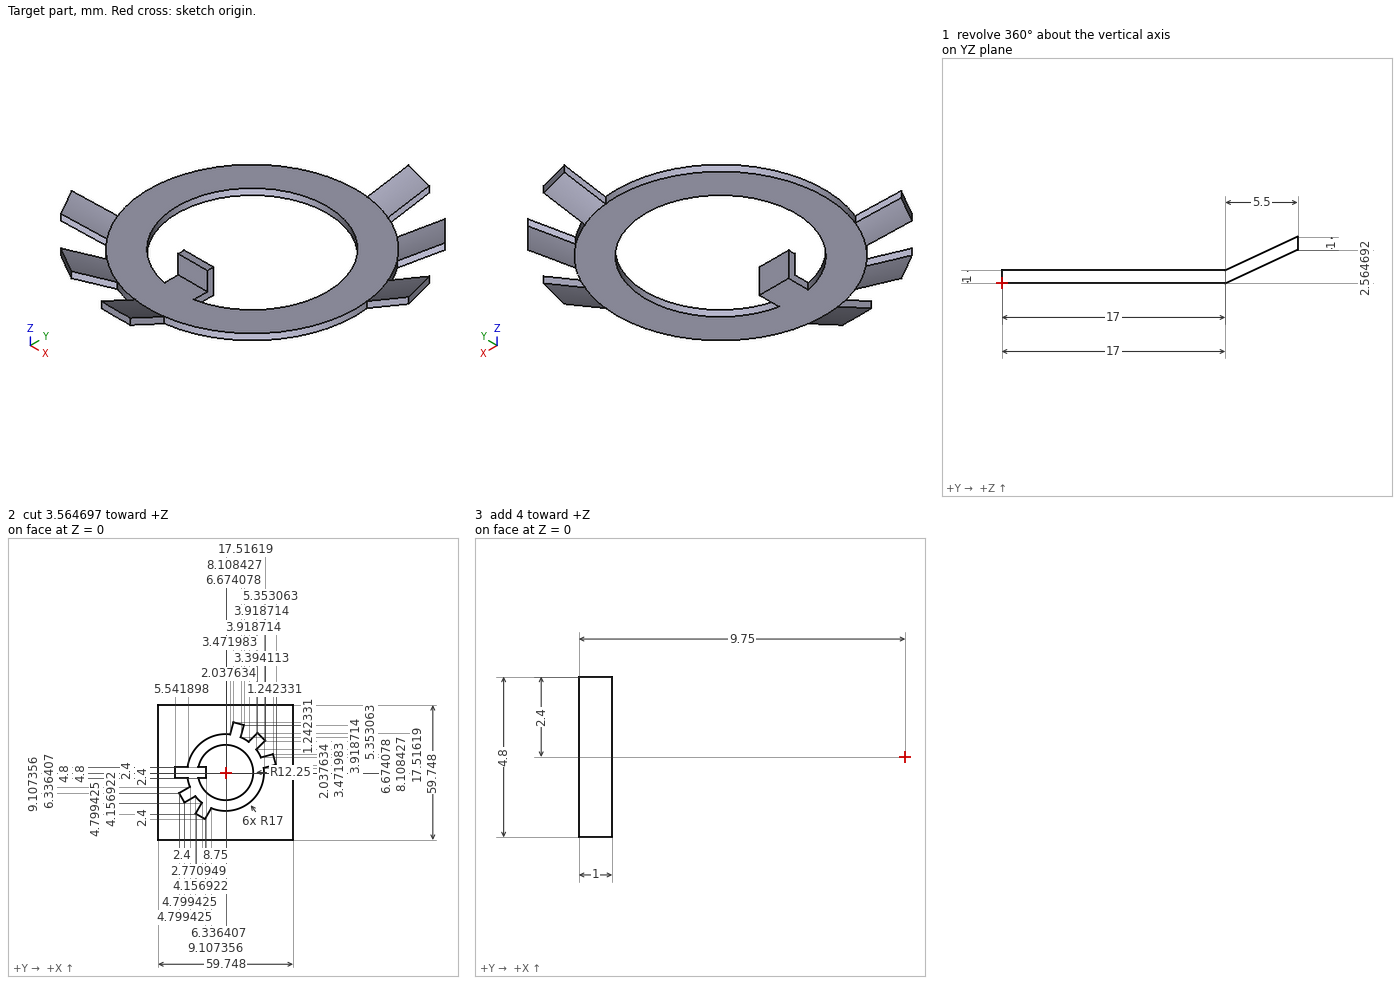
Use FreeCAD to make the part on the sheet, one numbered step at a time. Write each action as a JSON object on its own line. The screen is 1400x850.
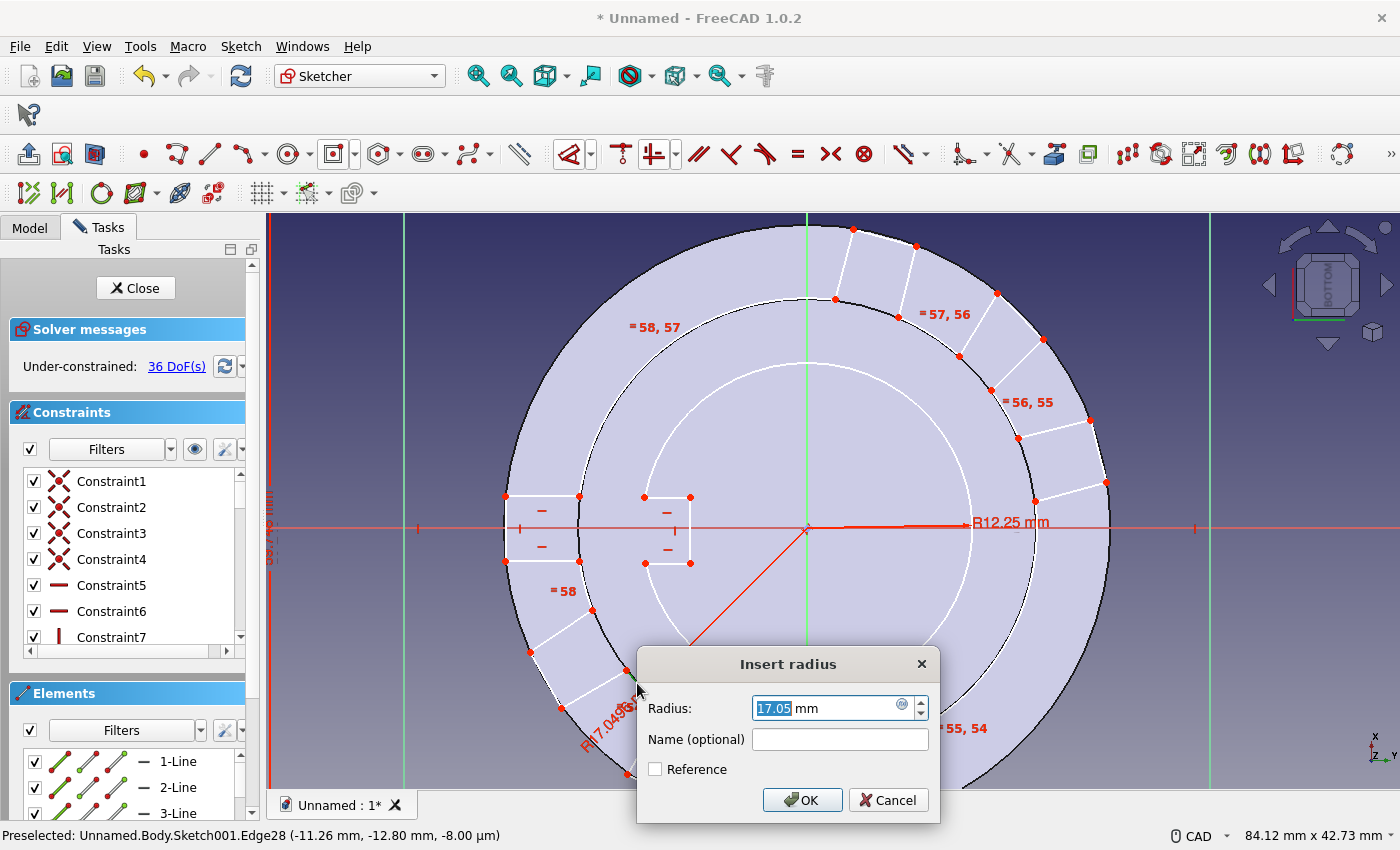
{"action": "type", "text": "17"}
{"action": "key", "text": "Return"}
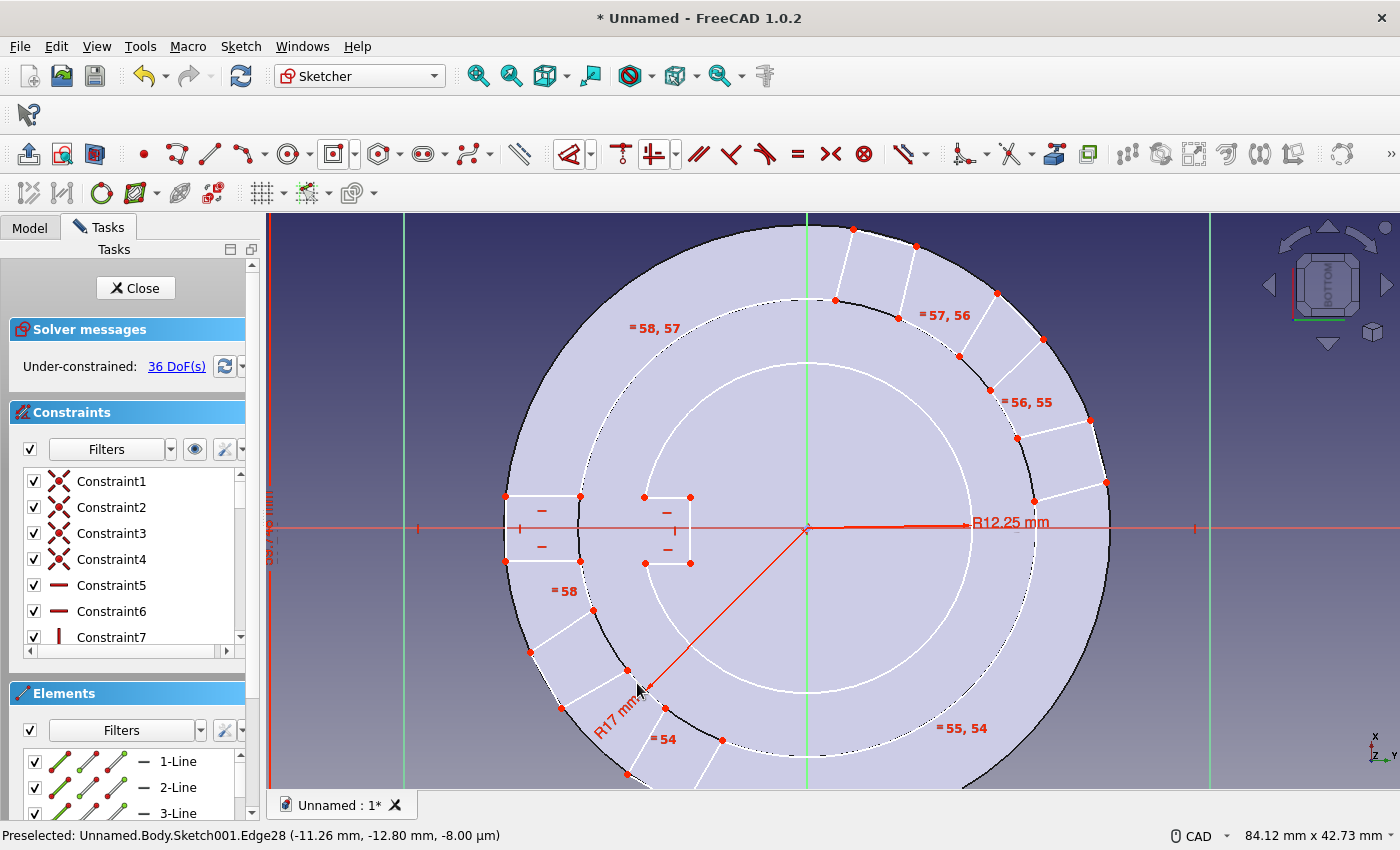
{"action": "left_click", "coordinate": [690, 544]}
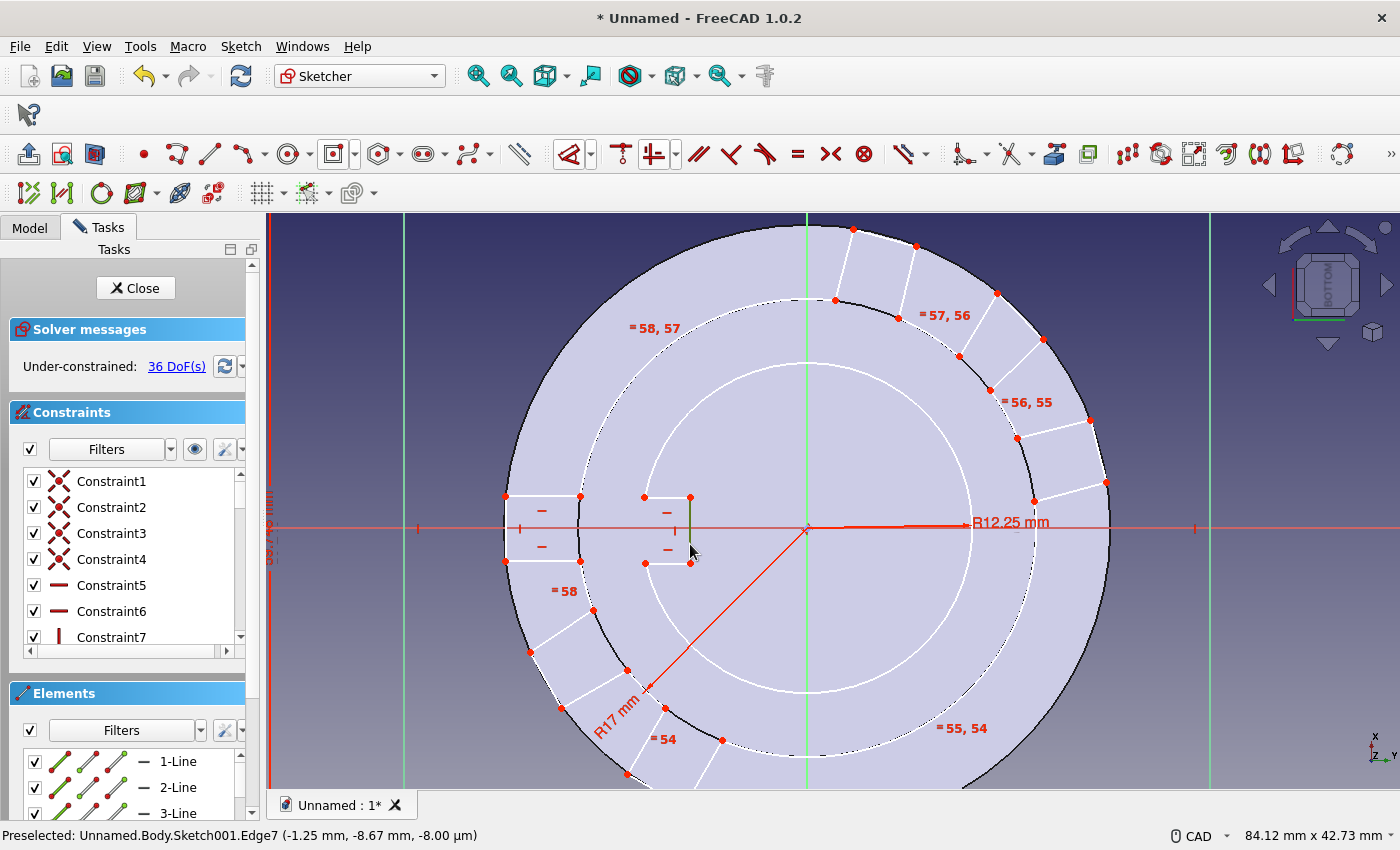
{"action": "left_click", "coordinate": [590, 154]}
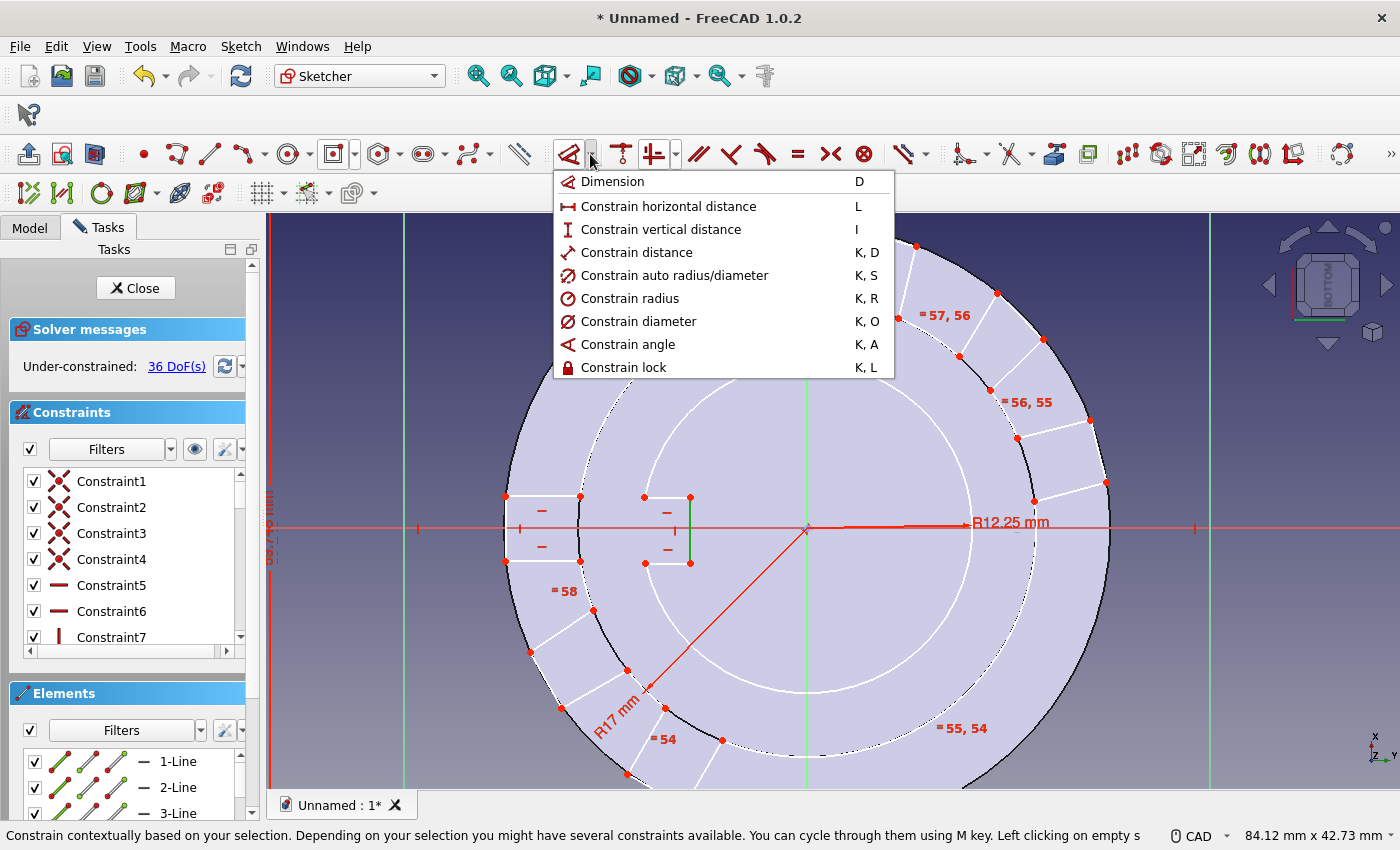
{"action": "left_click", "coordinate": [724, 230]}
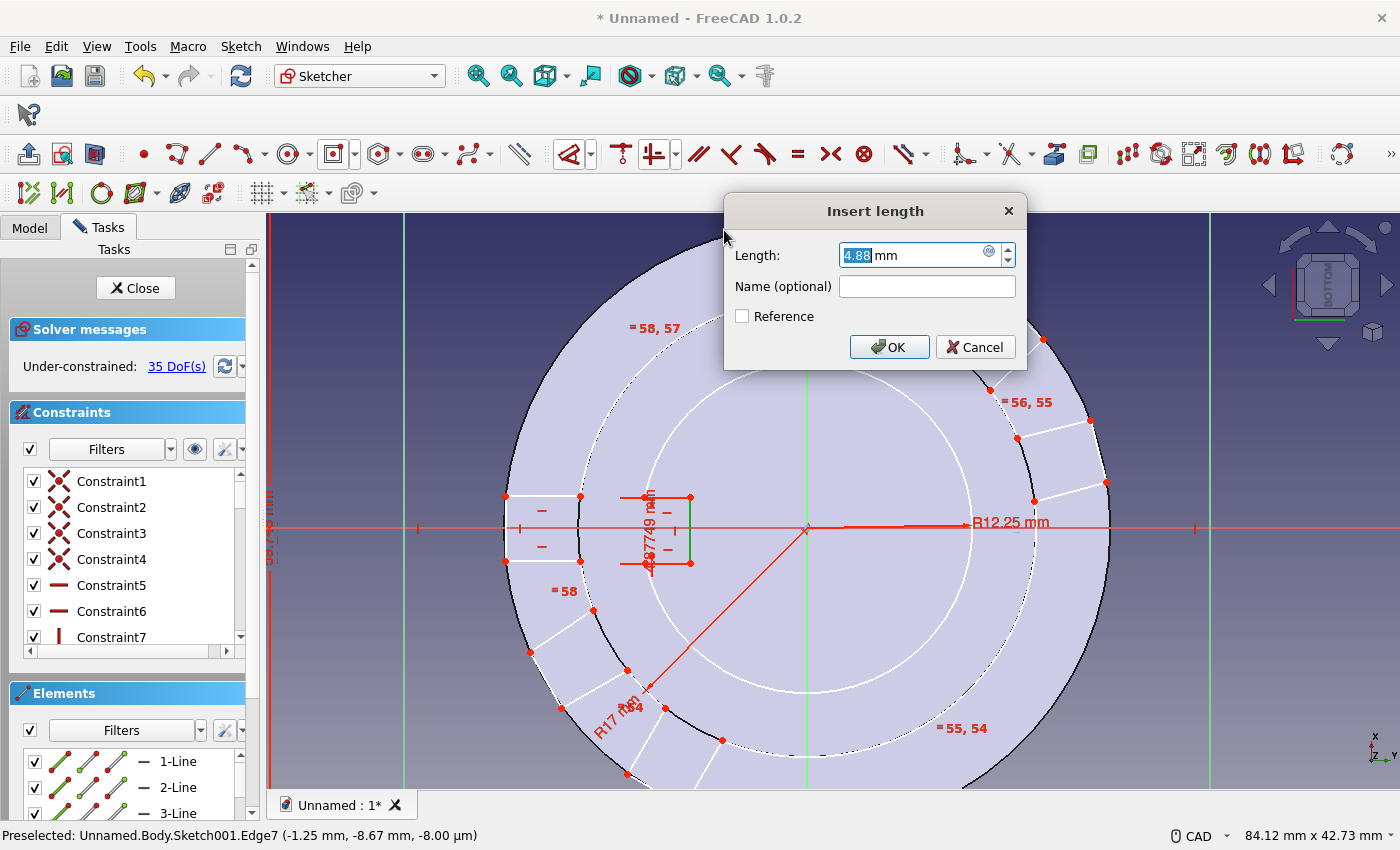
{"action": "type", "text": "4.8"}
{"action": "key", "text": "Return"}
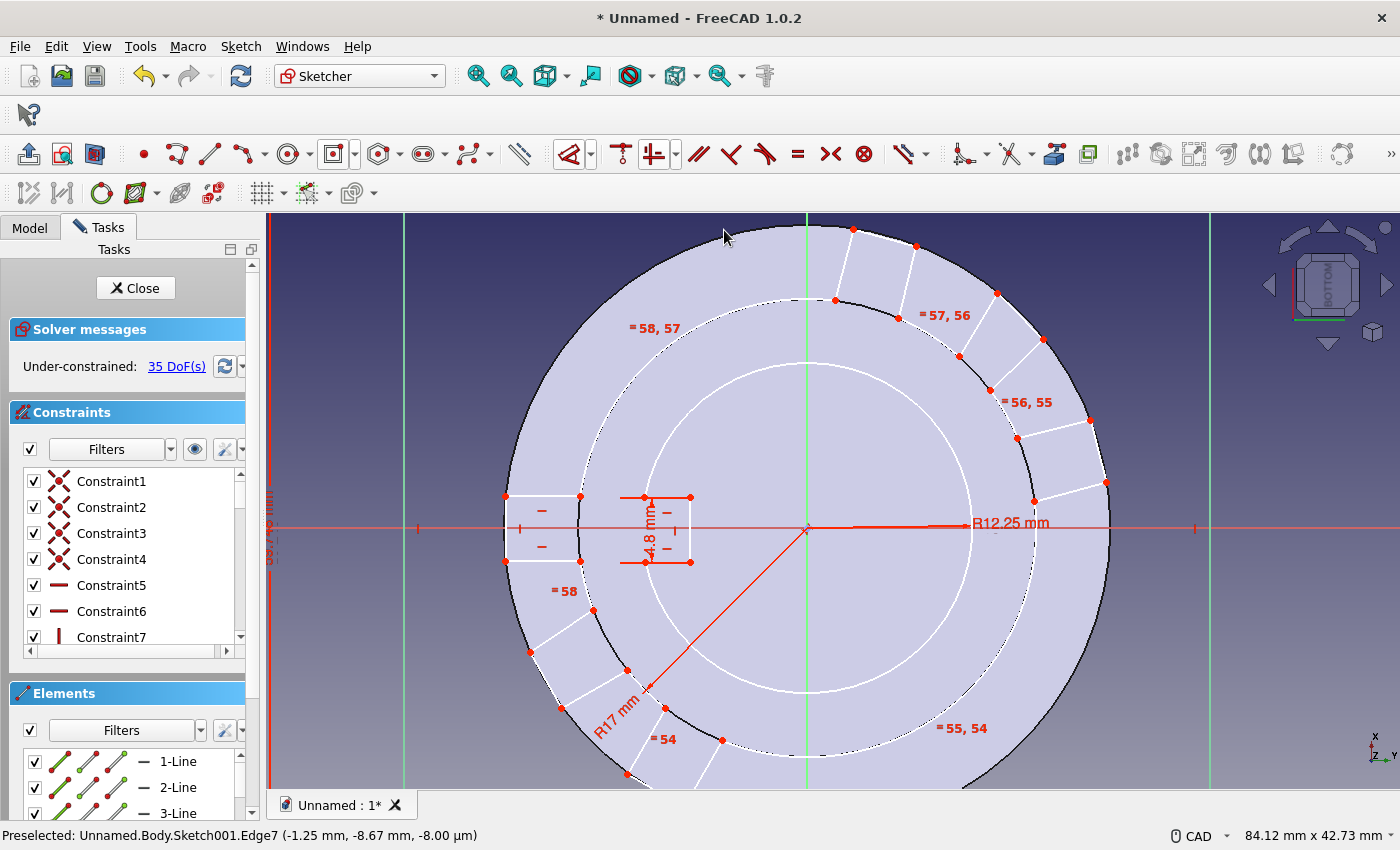
{"action": "left_click", "coordinate": [506, 516]}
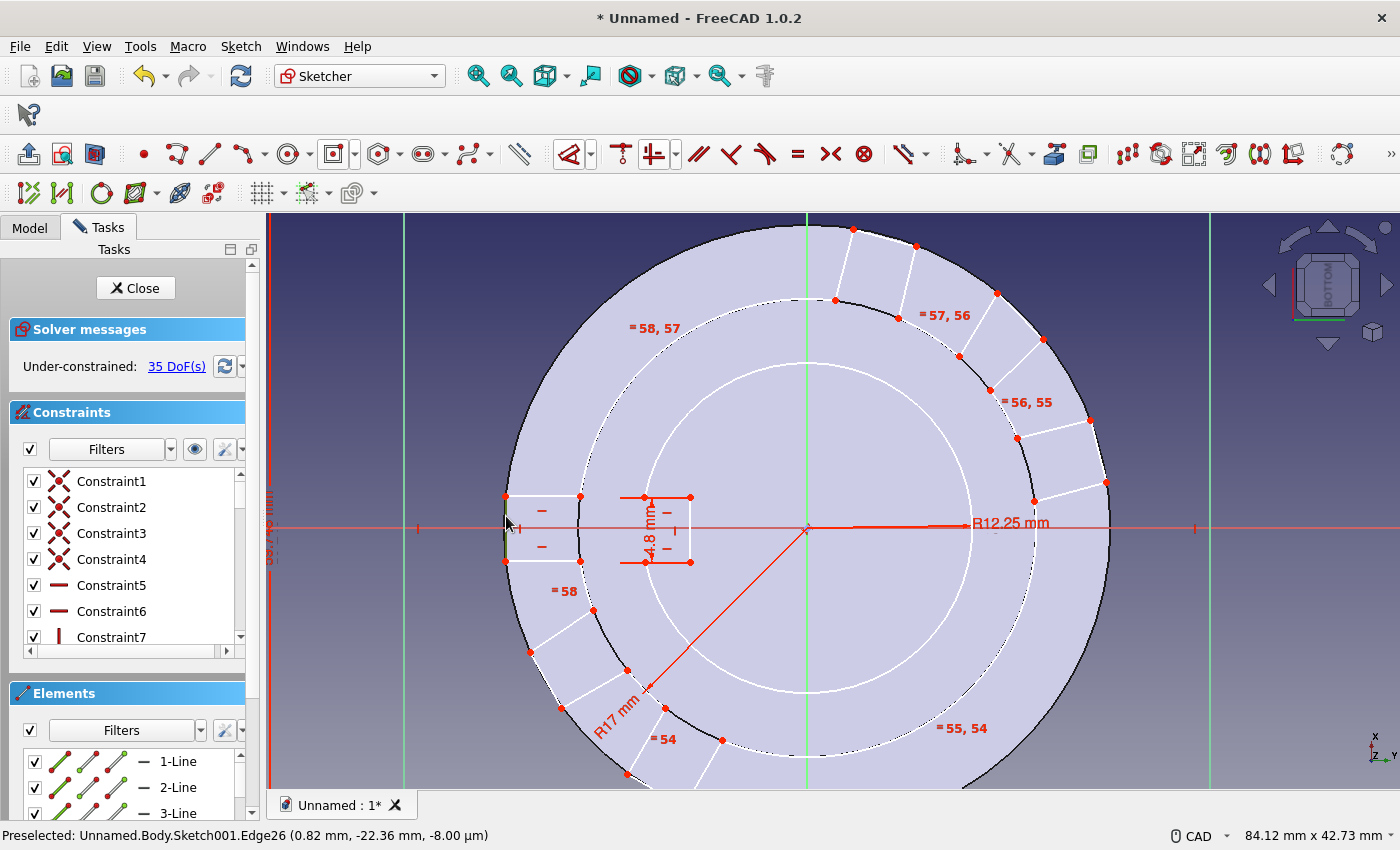
{"action": "left_click", "coordinate": [590, 154]}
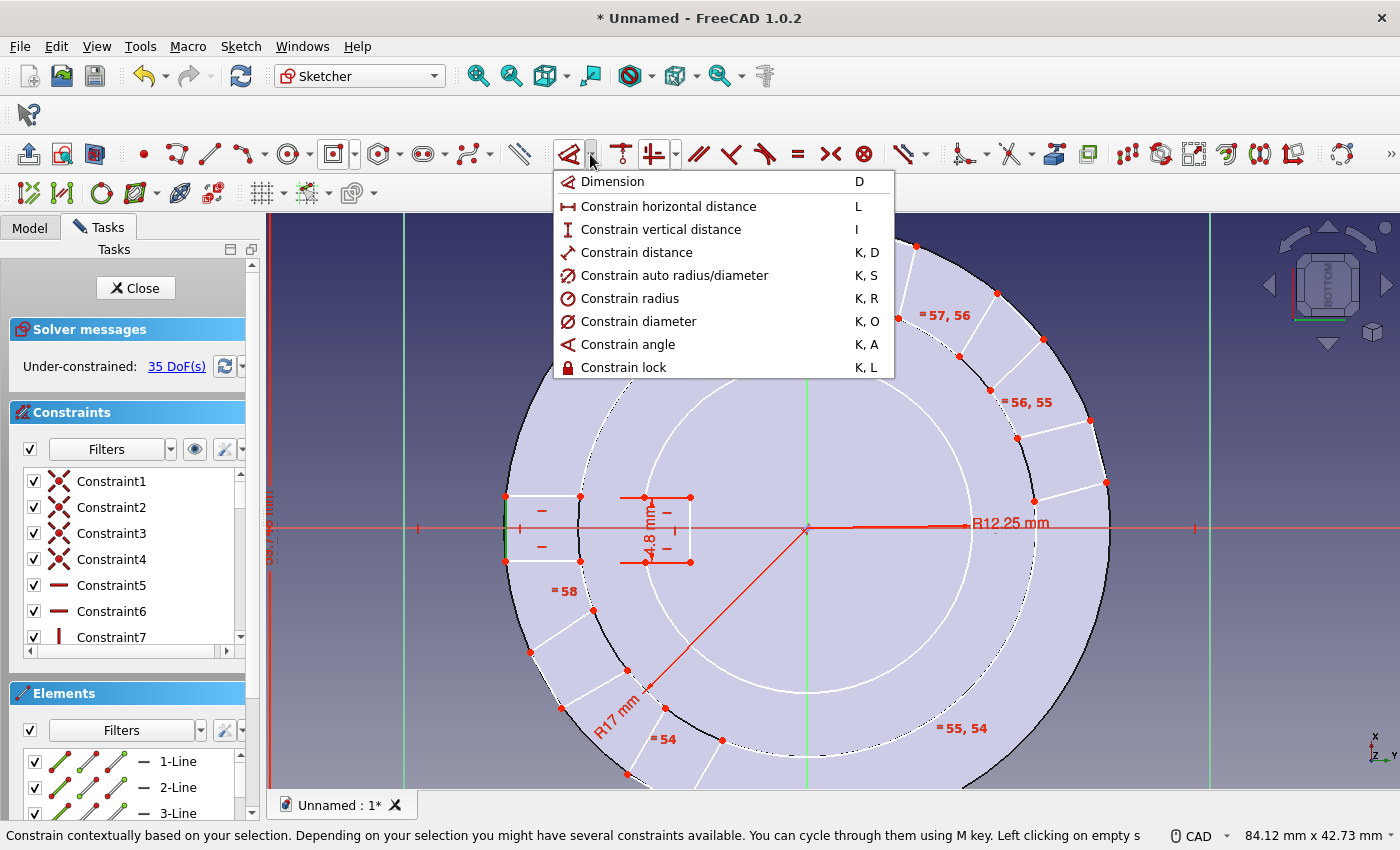
{"action": "left_click", "coordinate": [724, 230]}